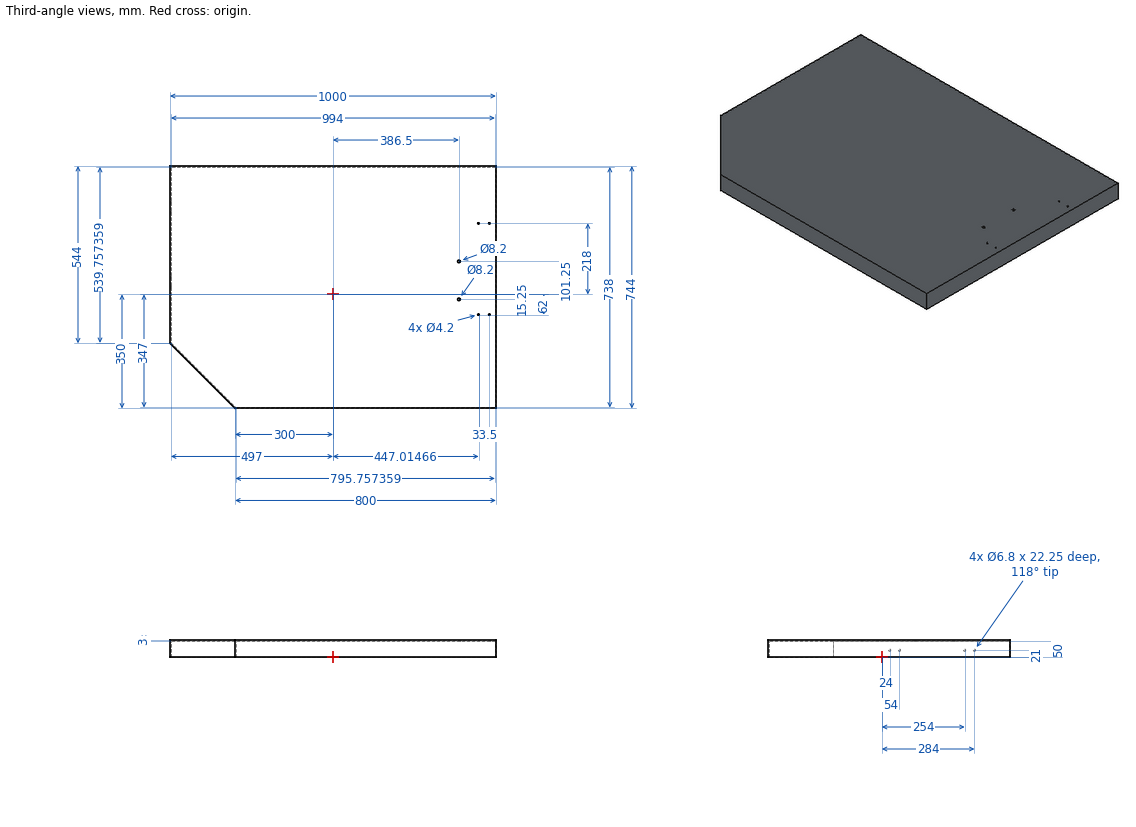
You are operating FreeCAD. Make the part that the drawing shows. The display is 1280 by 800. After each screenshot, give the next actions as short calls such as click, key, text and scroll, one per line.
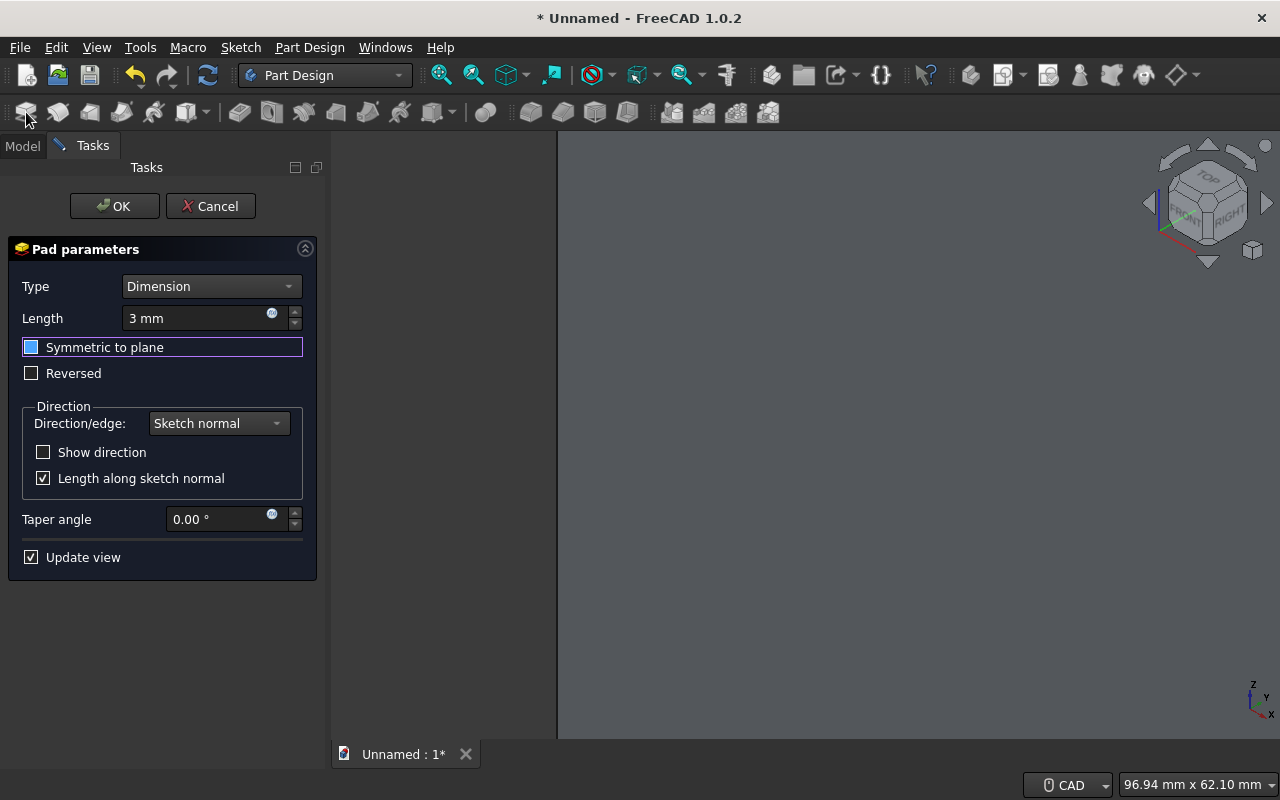
click(115, 206)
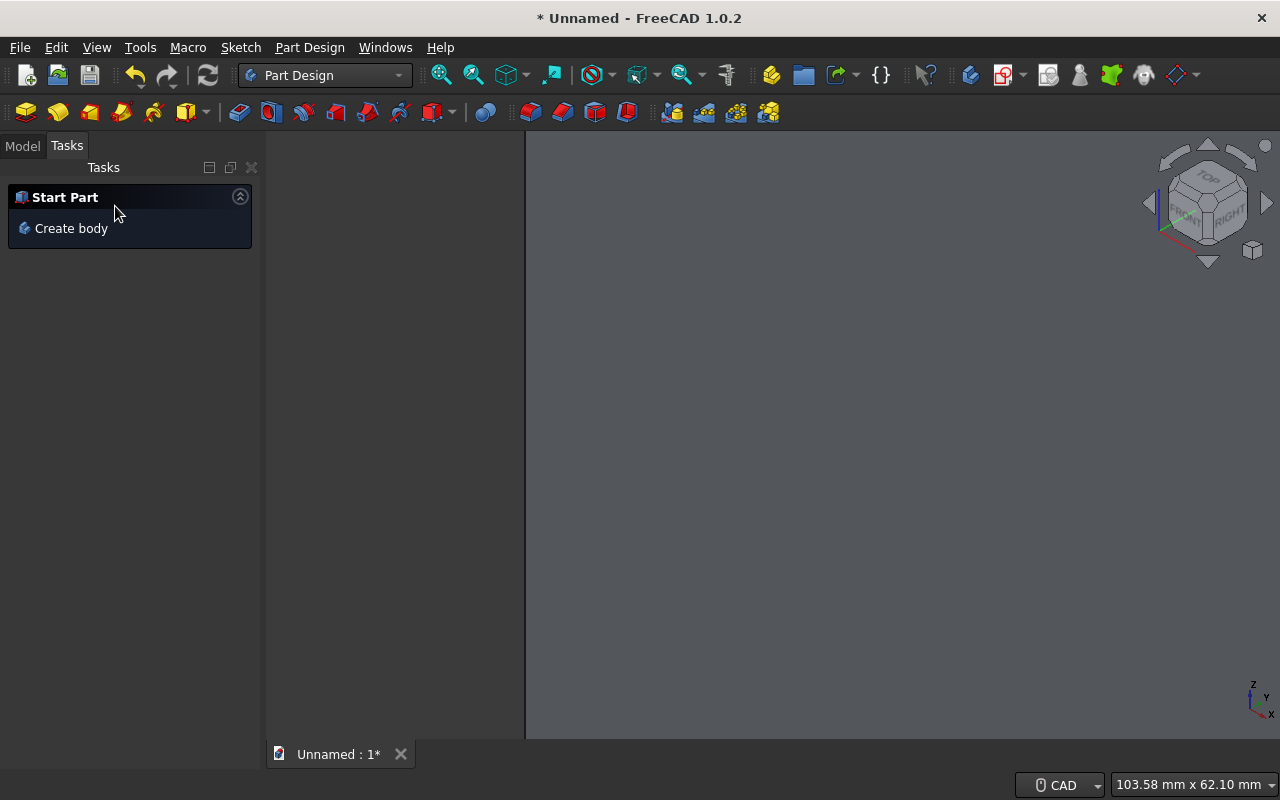
key(v)
key(f)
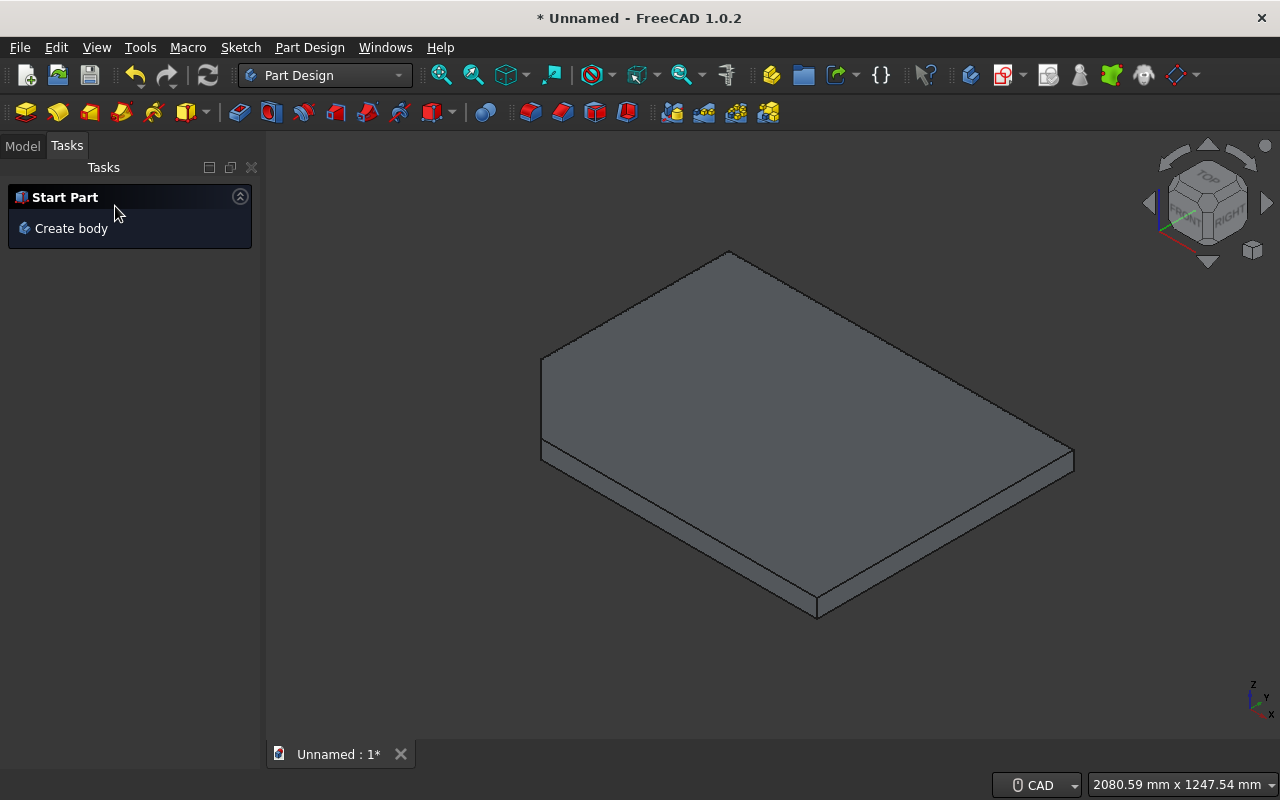
click(773, 423)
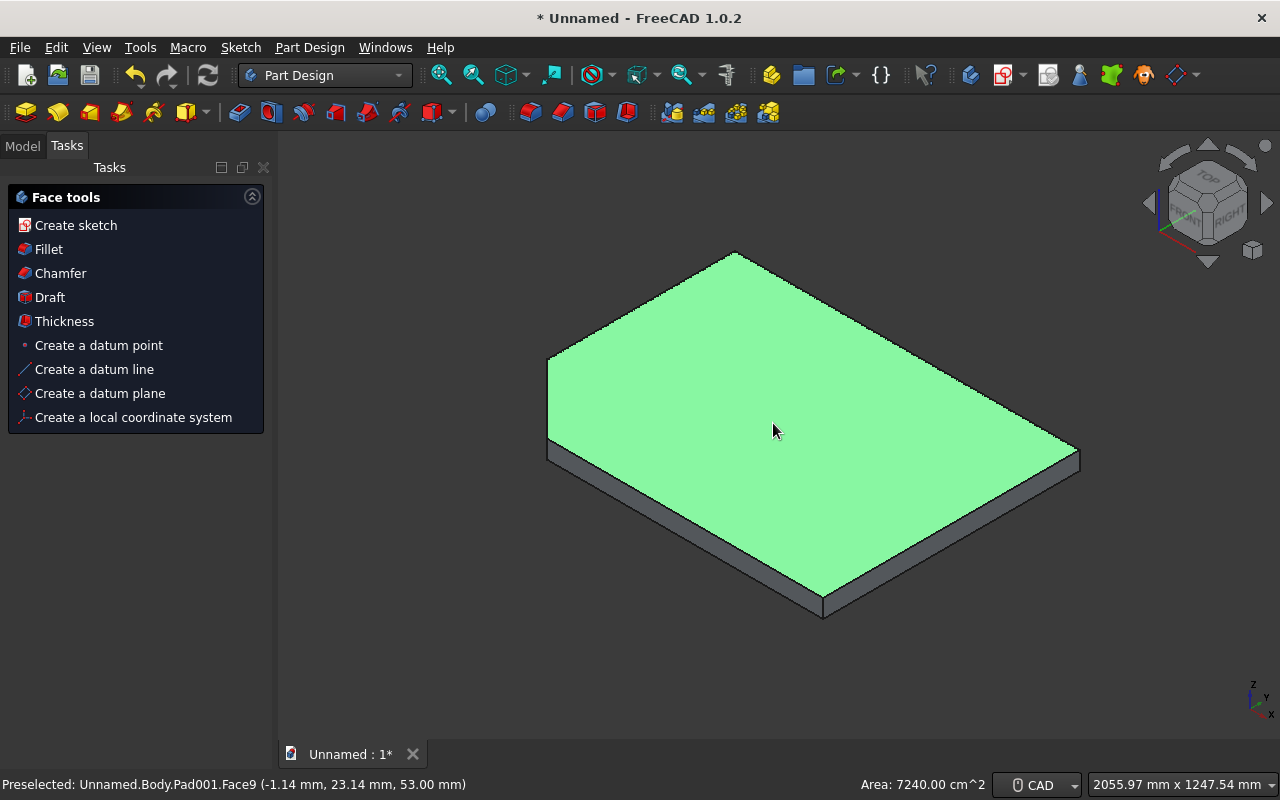
click(1004, 76)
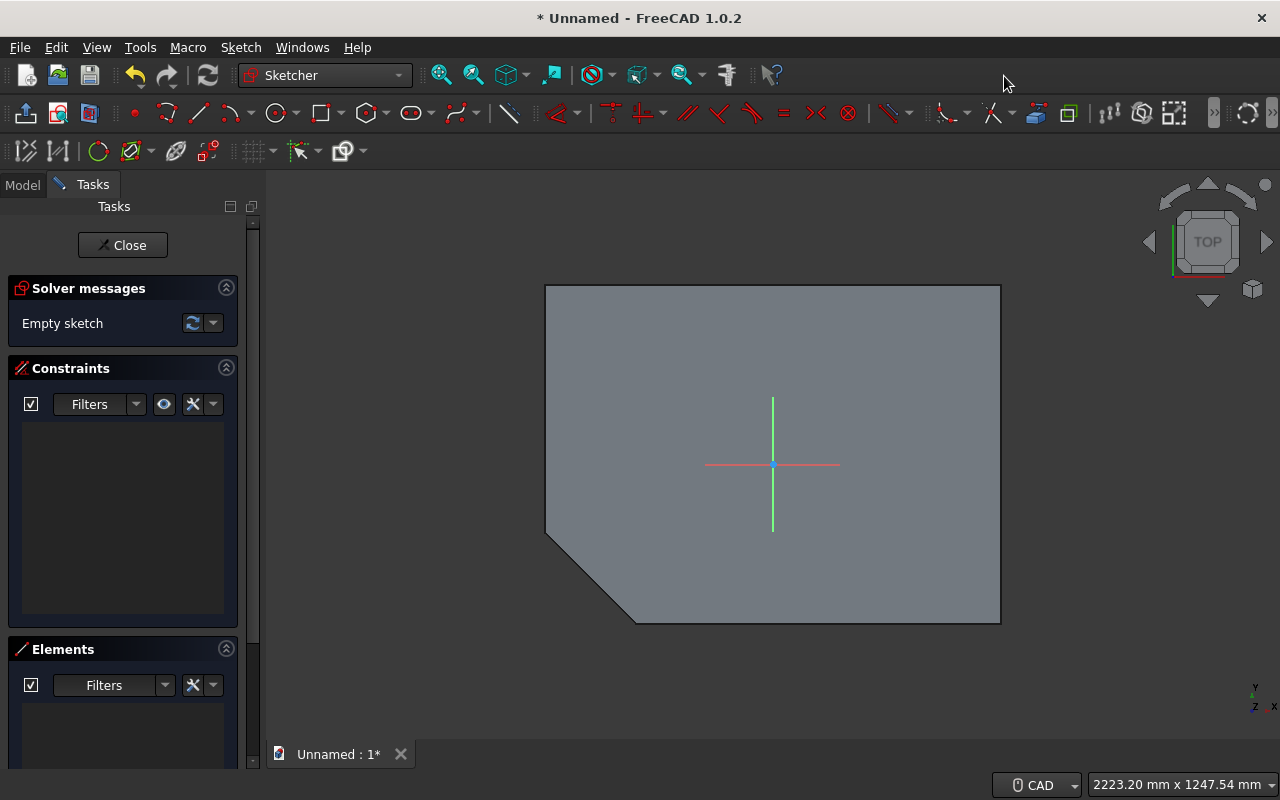
scroll(962, 416, up, 15)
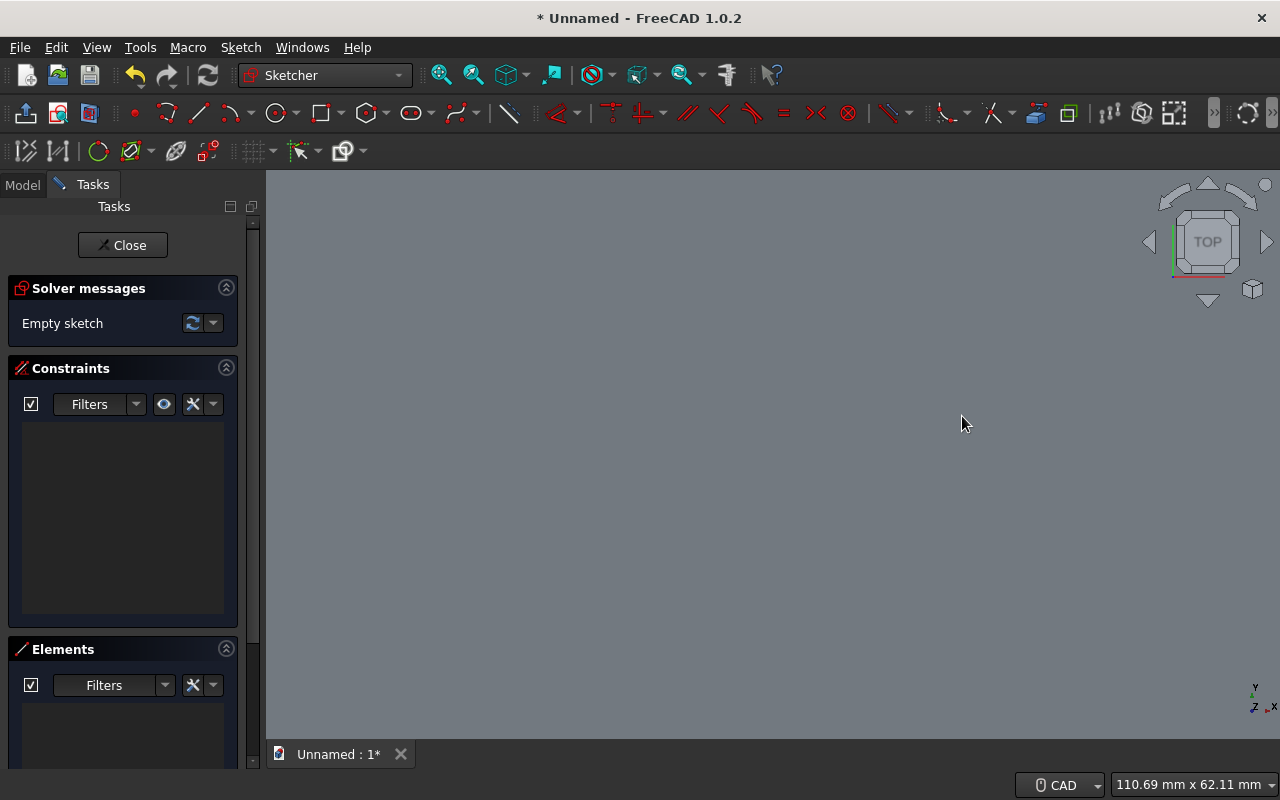
scroll(691, 455, up, 8)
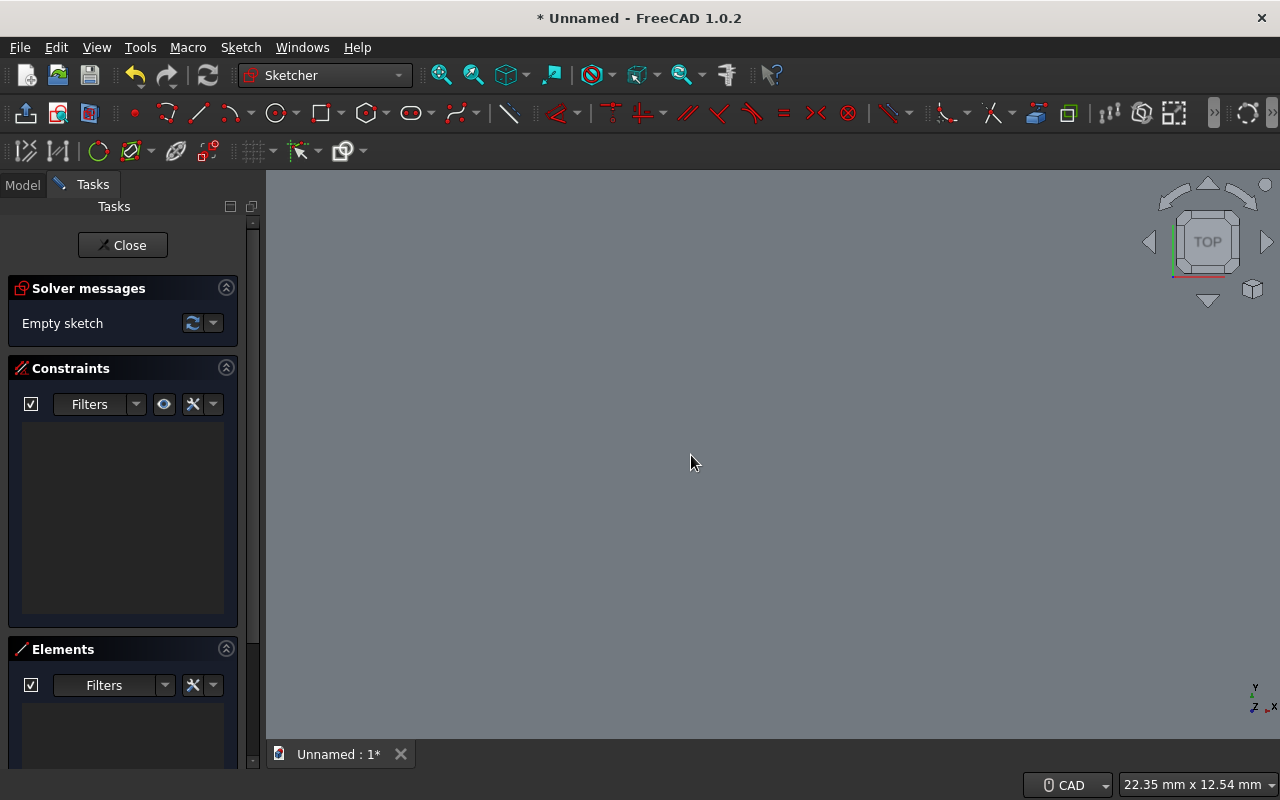
click(276, 114)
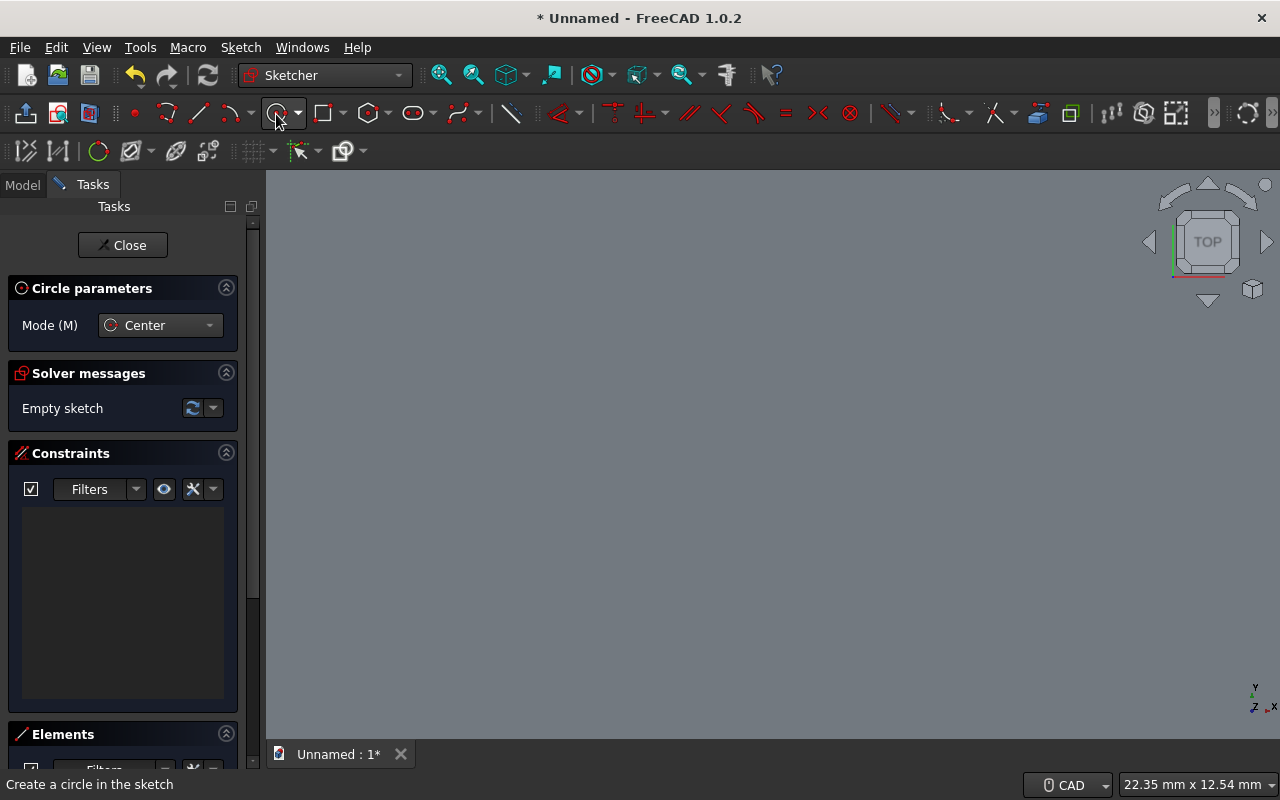
click(701, 453)
move(833, 322)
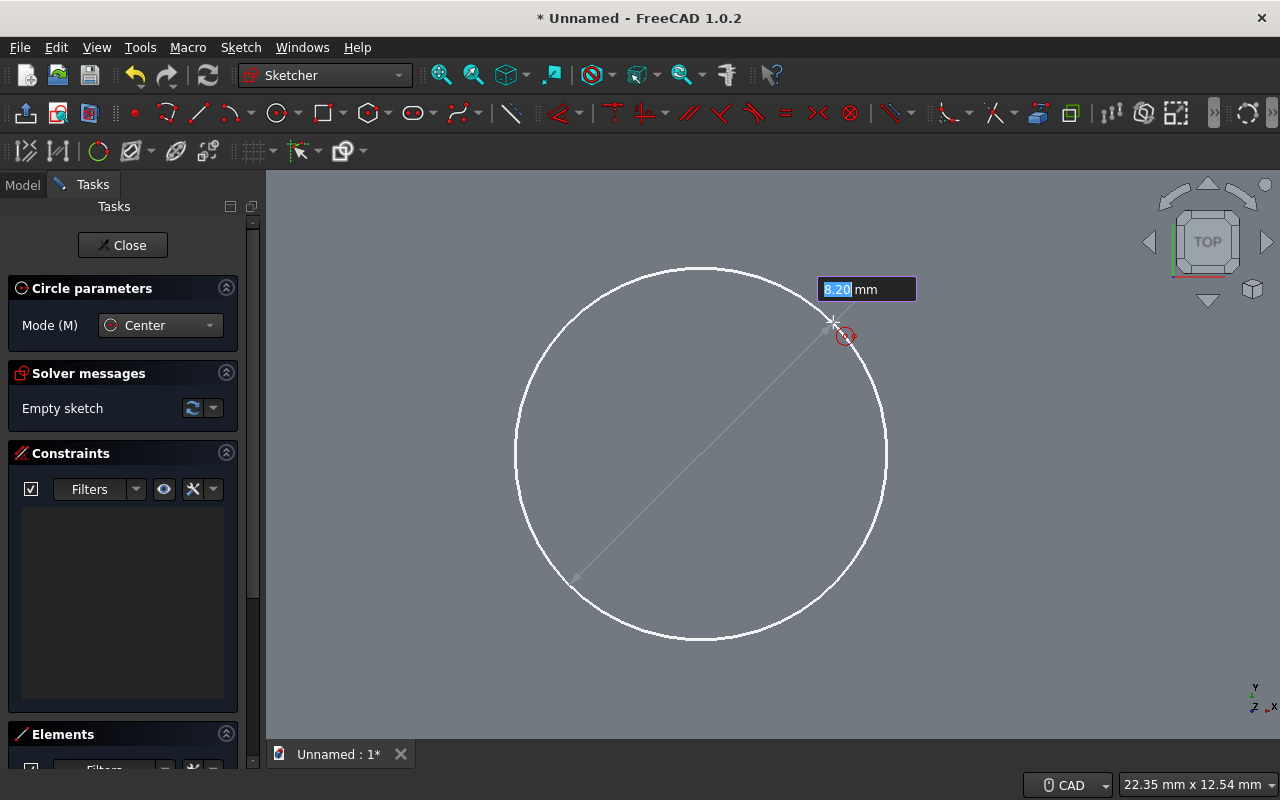
text(8.2)
key(Return)
key(Escape)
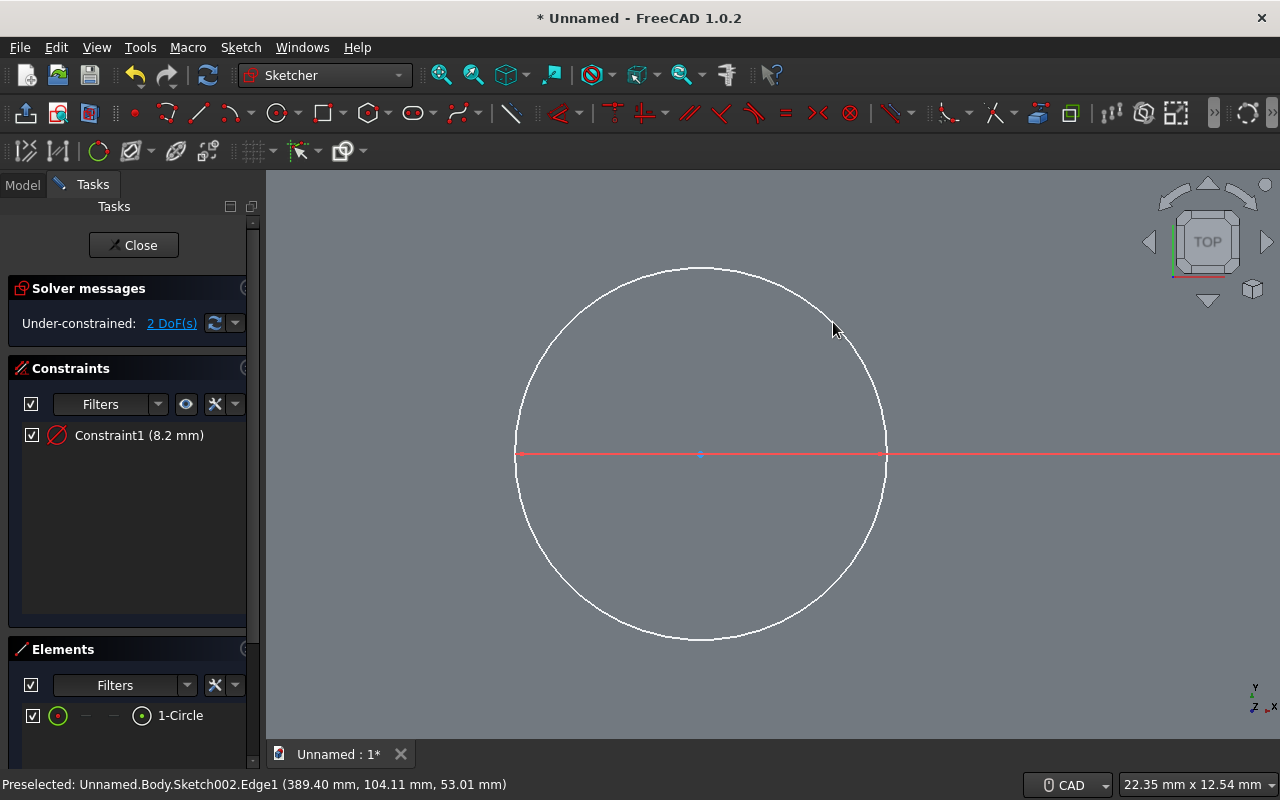
click(558, 114)